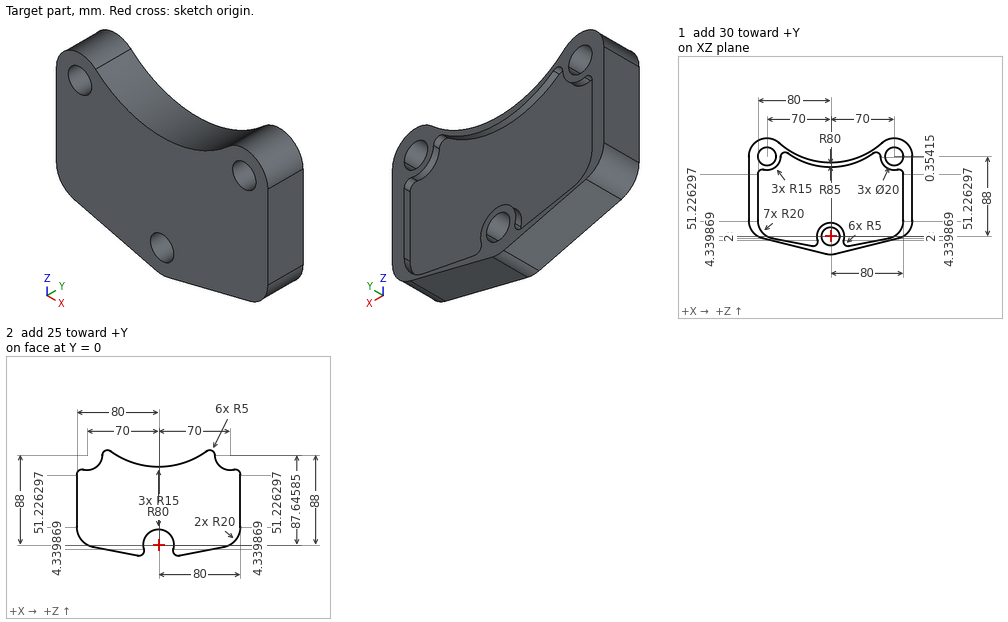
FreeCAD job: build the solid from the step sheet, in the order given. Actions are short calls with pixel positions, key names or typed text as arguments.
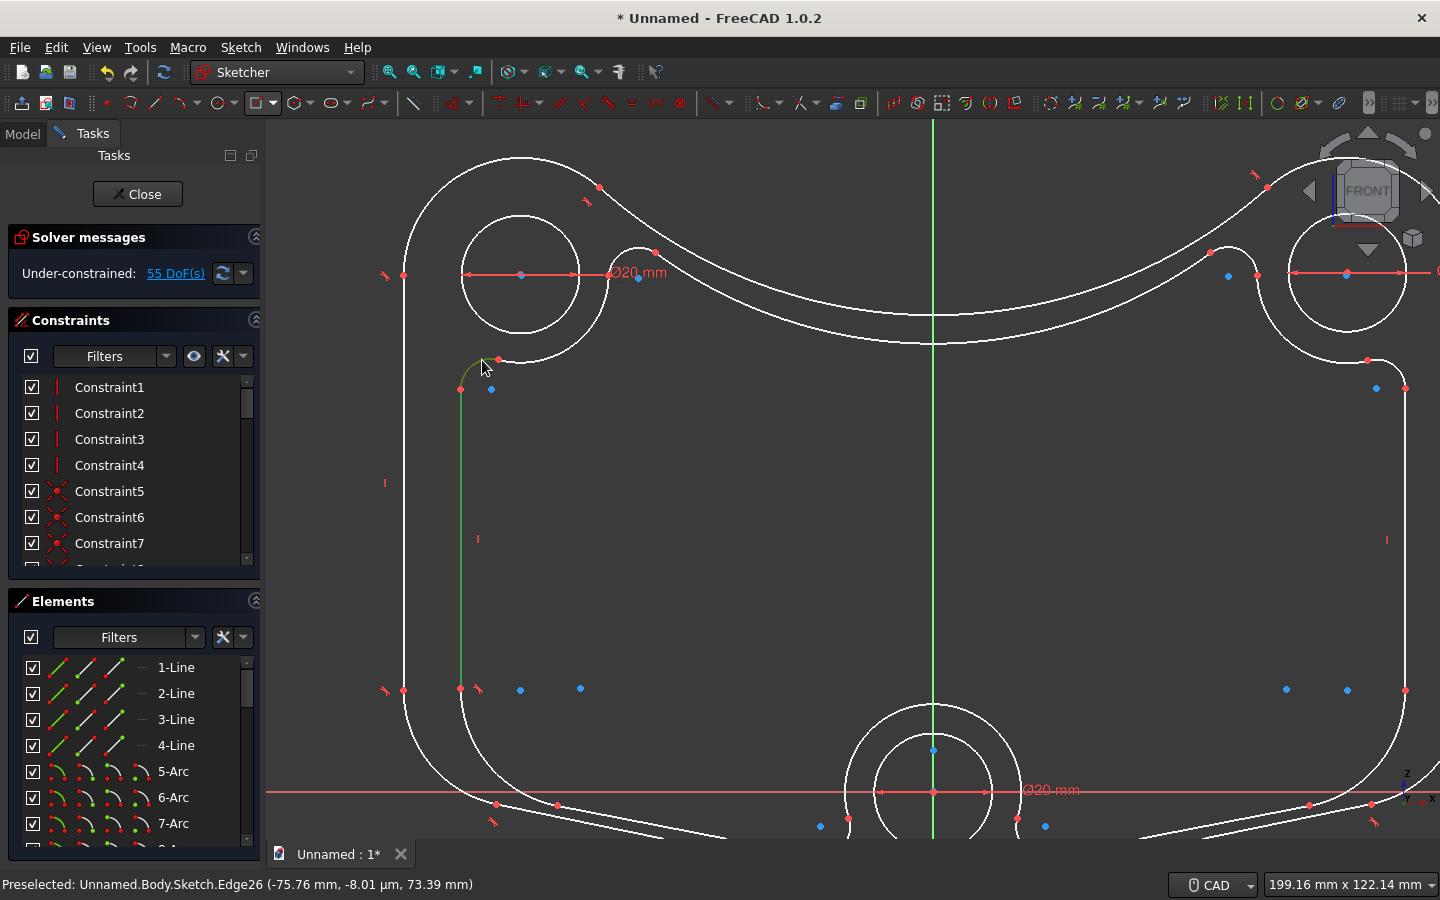
click(608, 104)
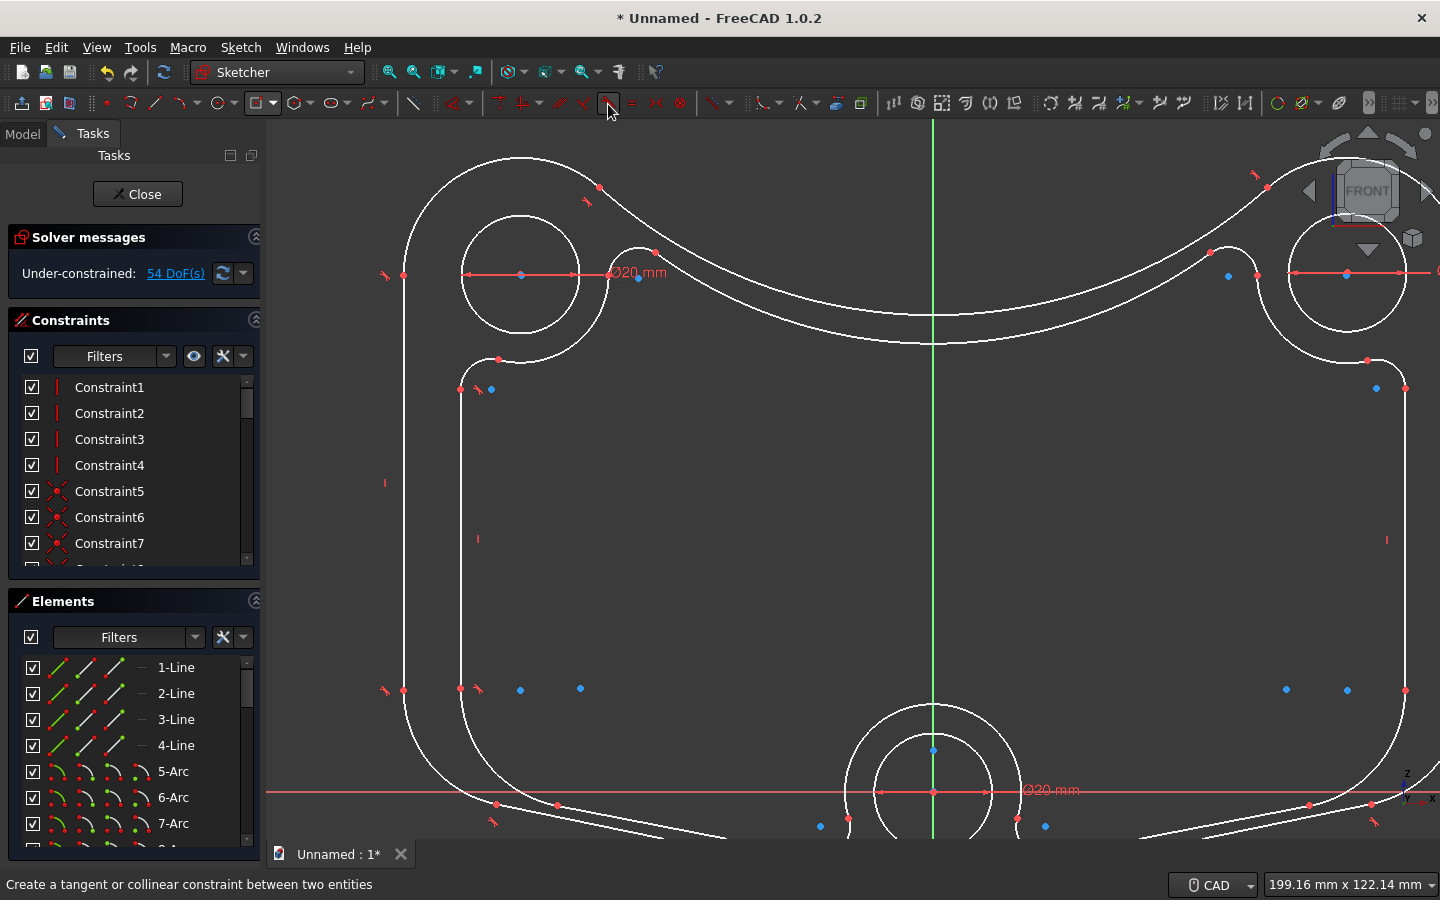
scroll(482, 360, down, 2)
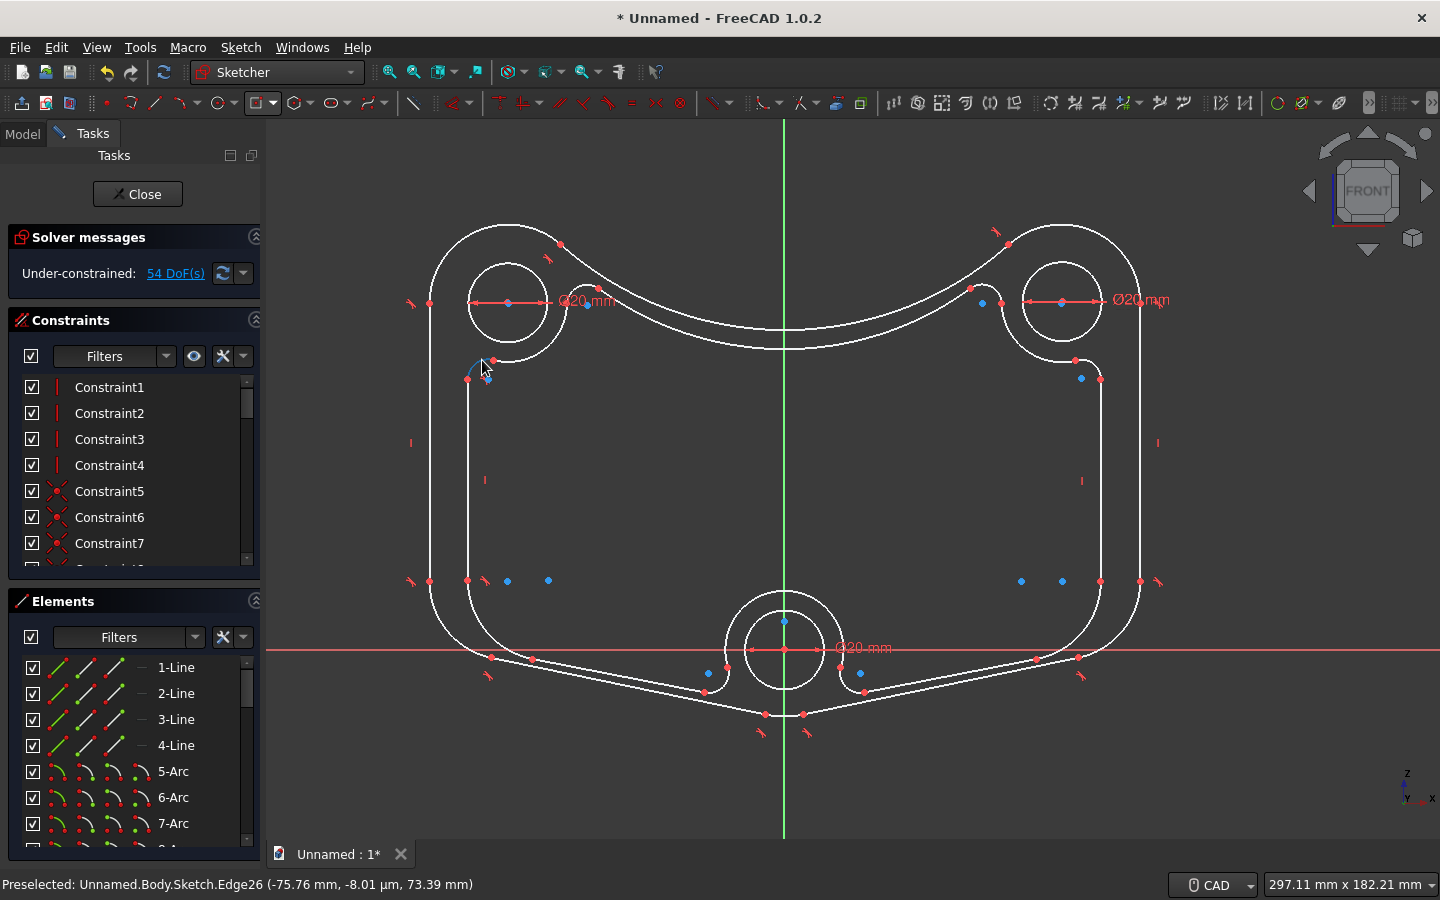
scroll(584, 669, up, 3)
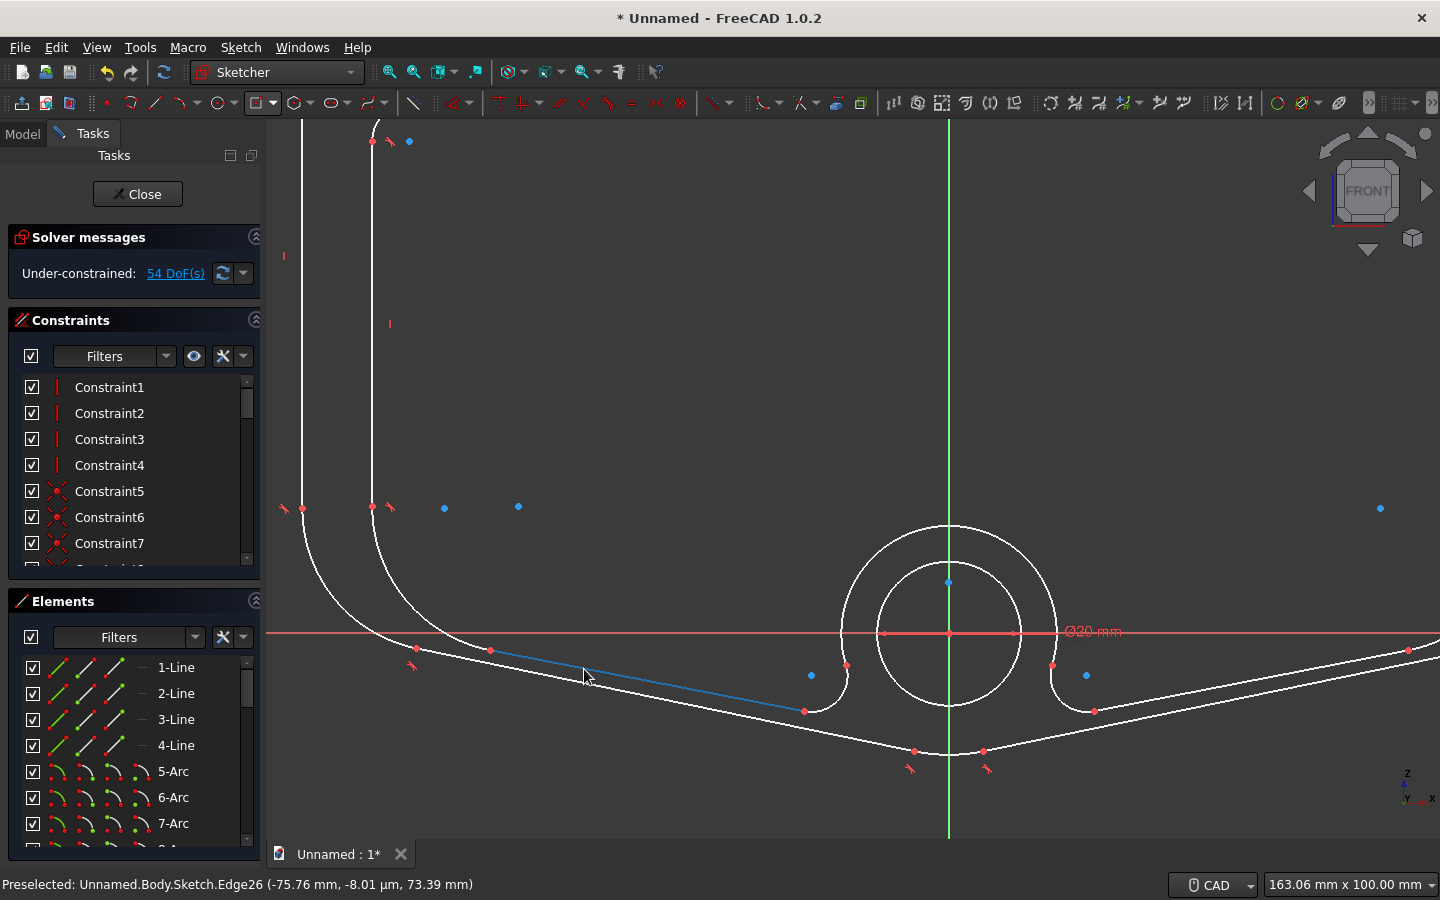
click(584, 669)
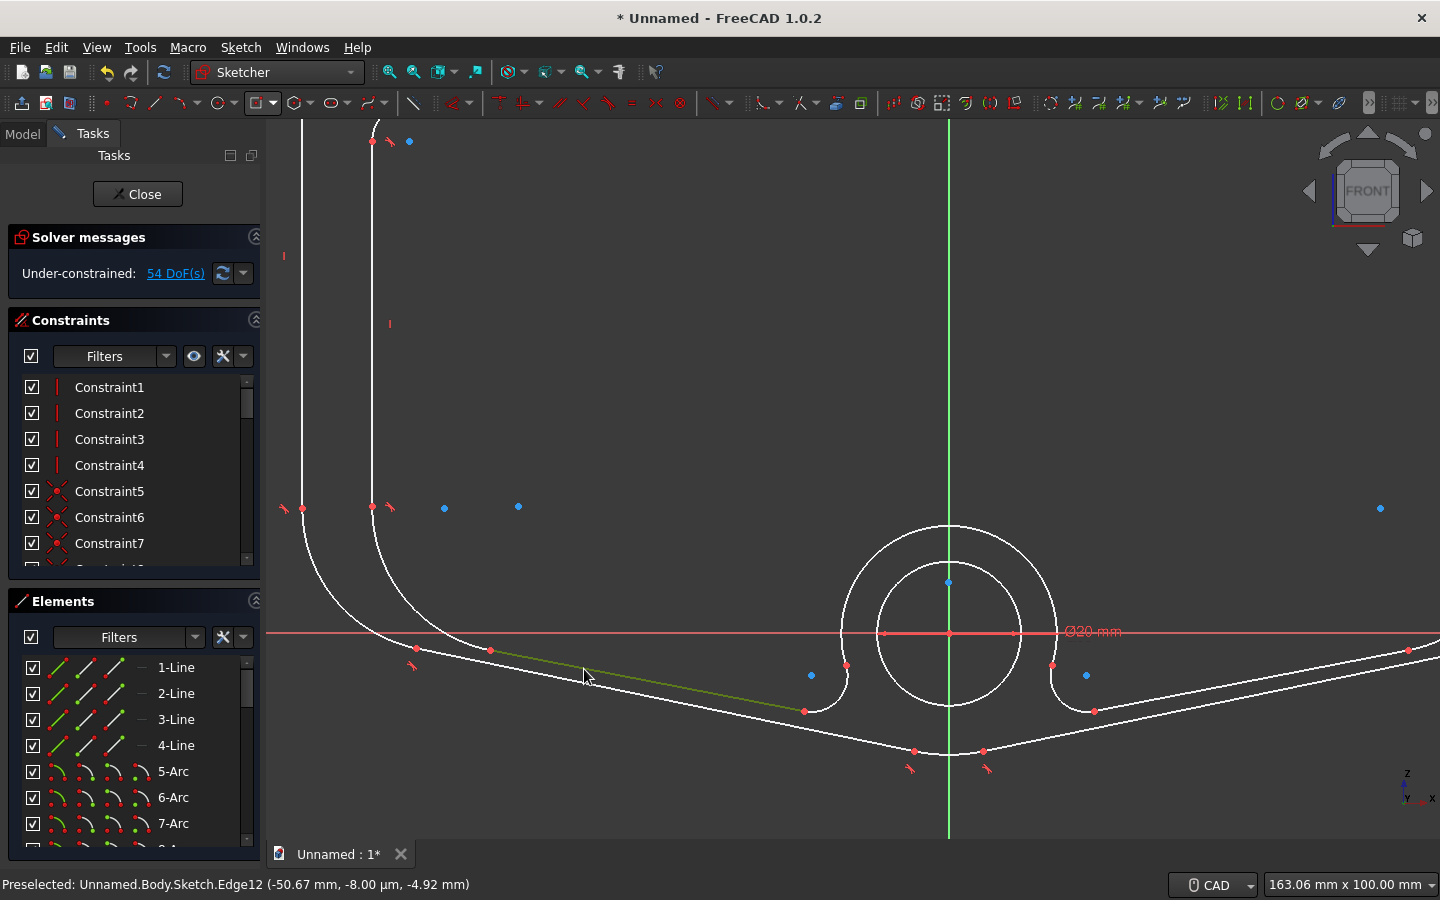
click(384, 565)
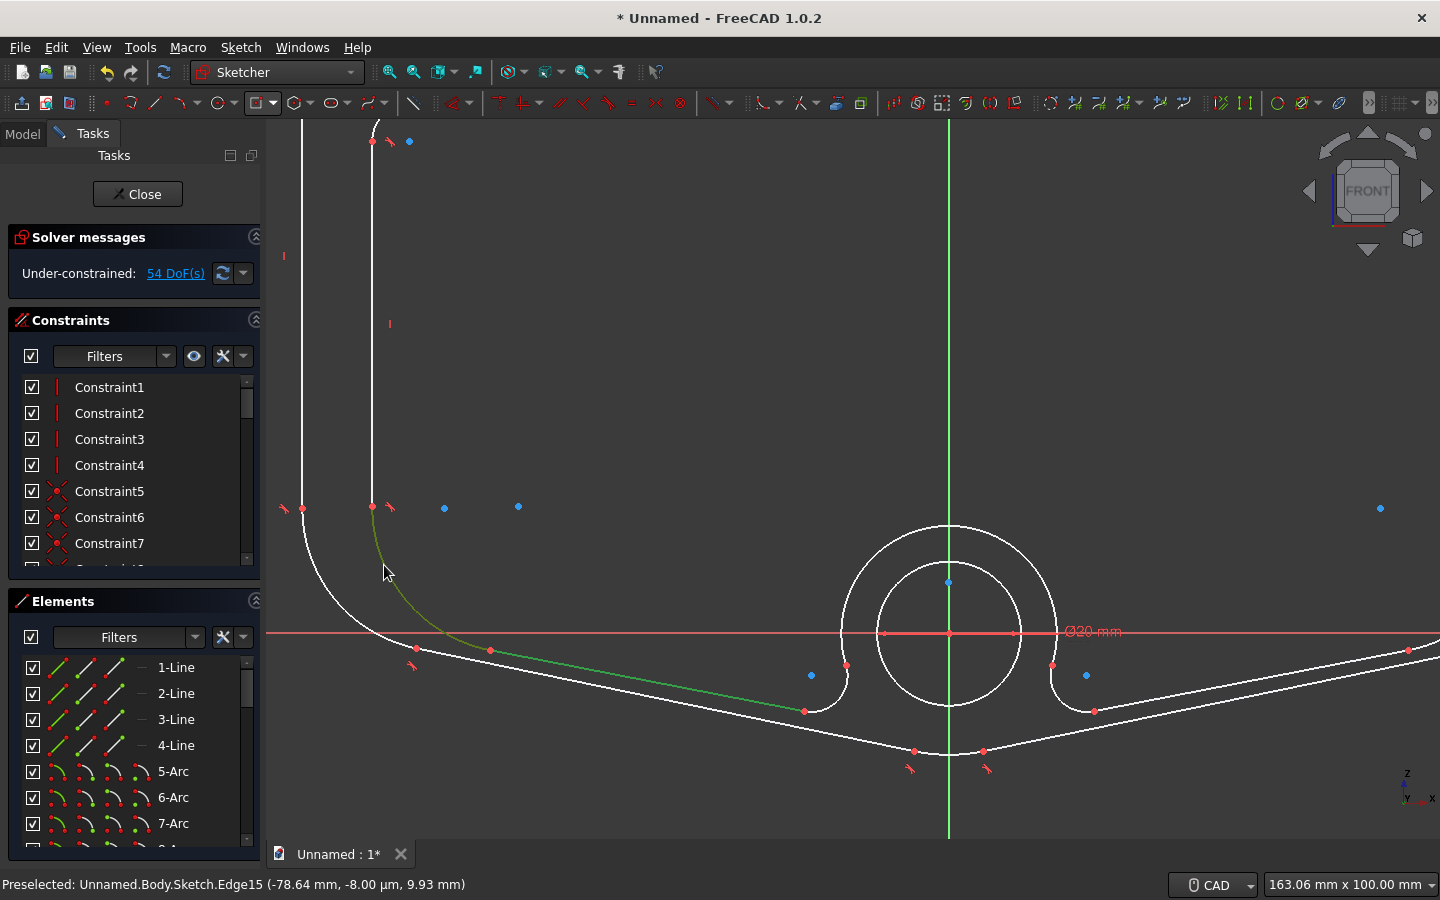
click(608, 104)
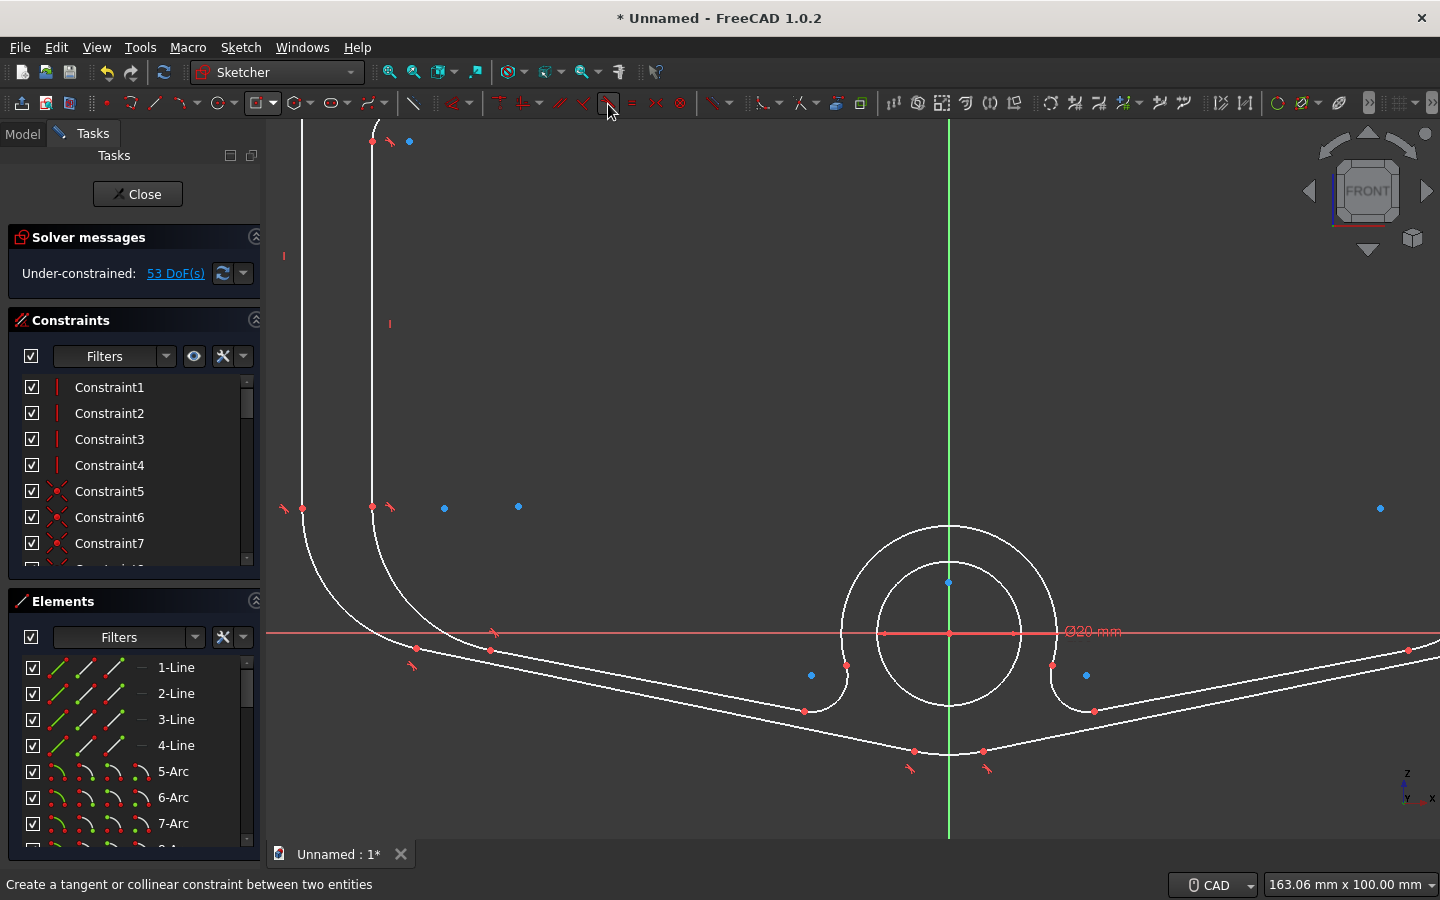
click(585, 669)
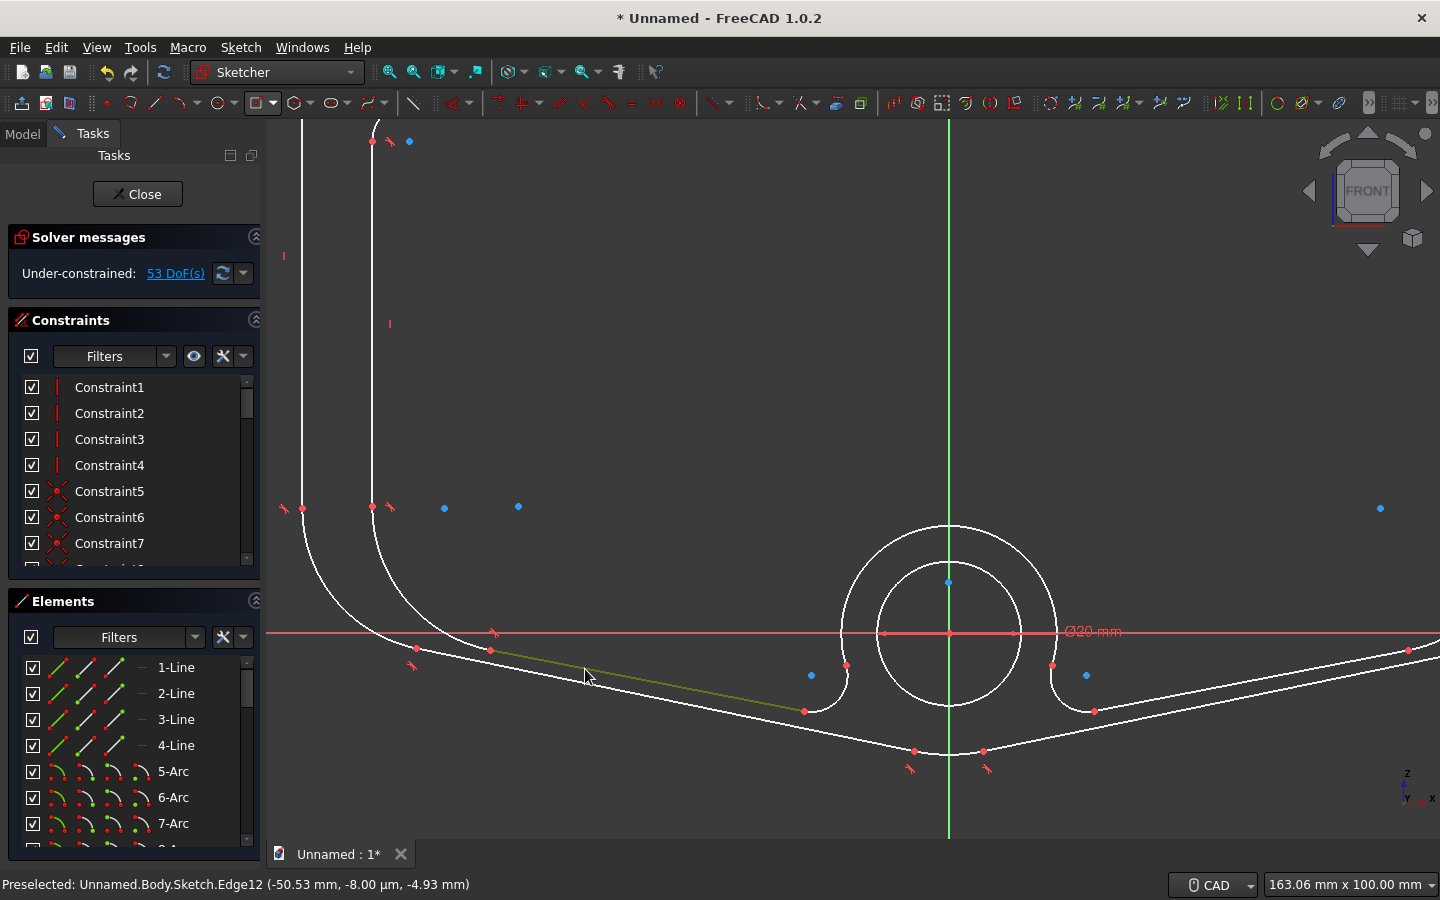
click(826, 709)